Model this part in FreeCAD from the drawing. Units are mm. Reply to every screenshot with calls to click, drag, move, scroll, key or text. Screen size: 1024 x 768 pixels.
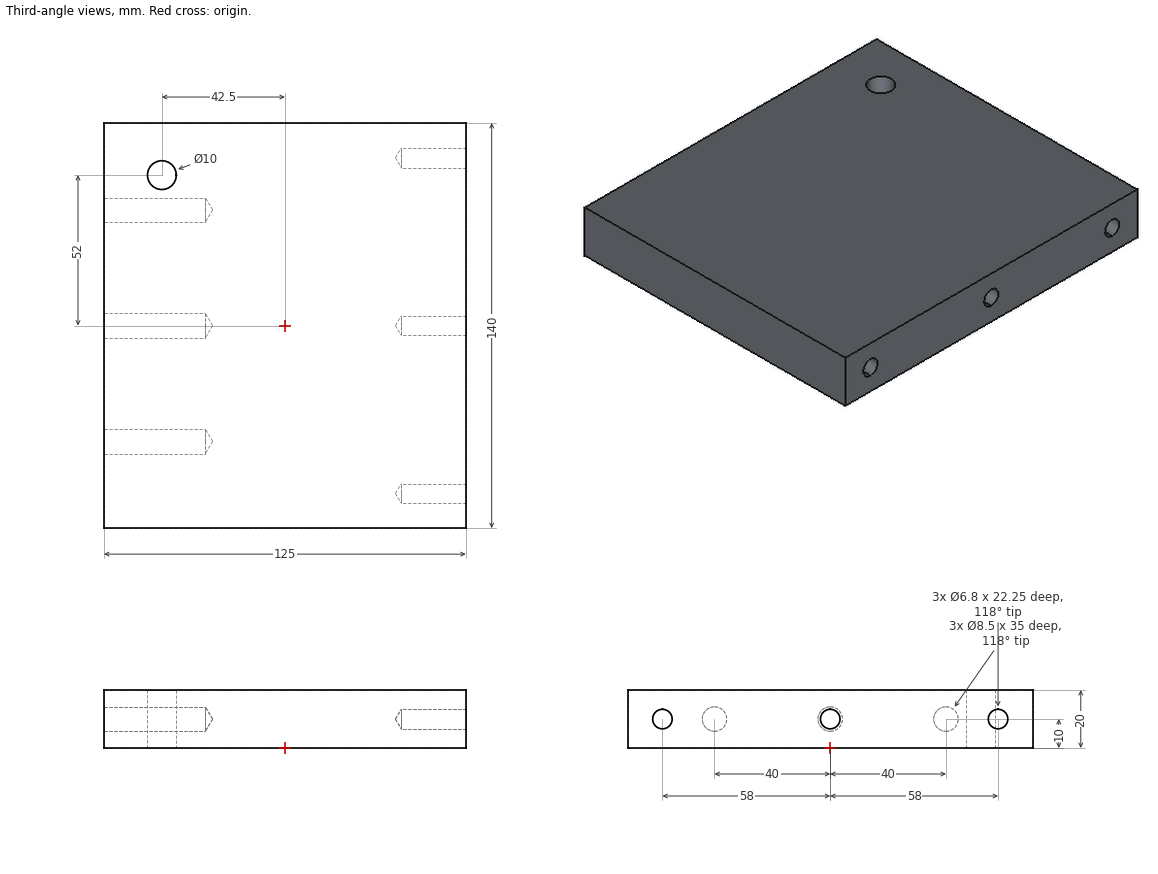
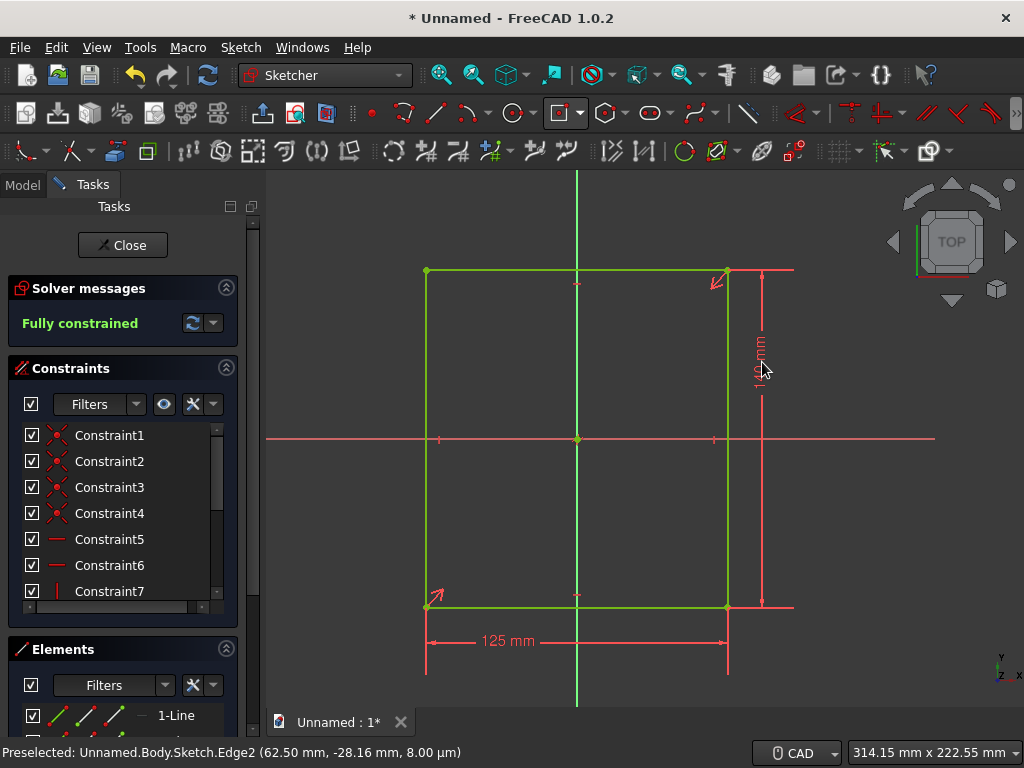
click(123, 245)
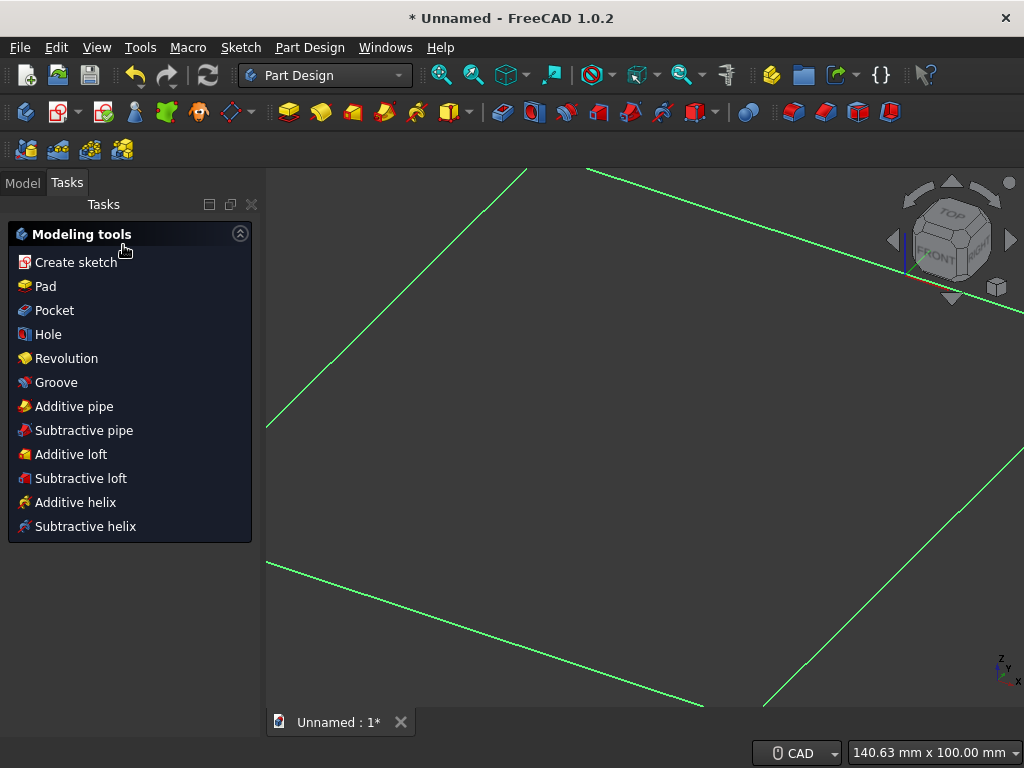
click(290, 112)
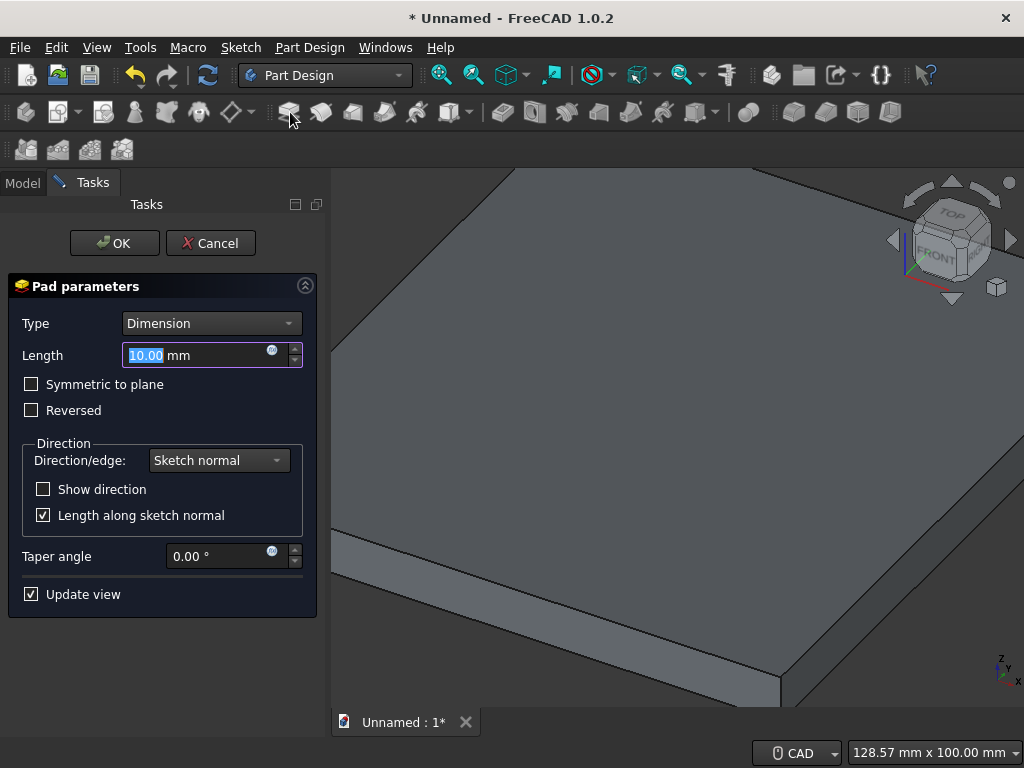
text(20)
key(Tab)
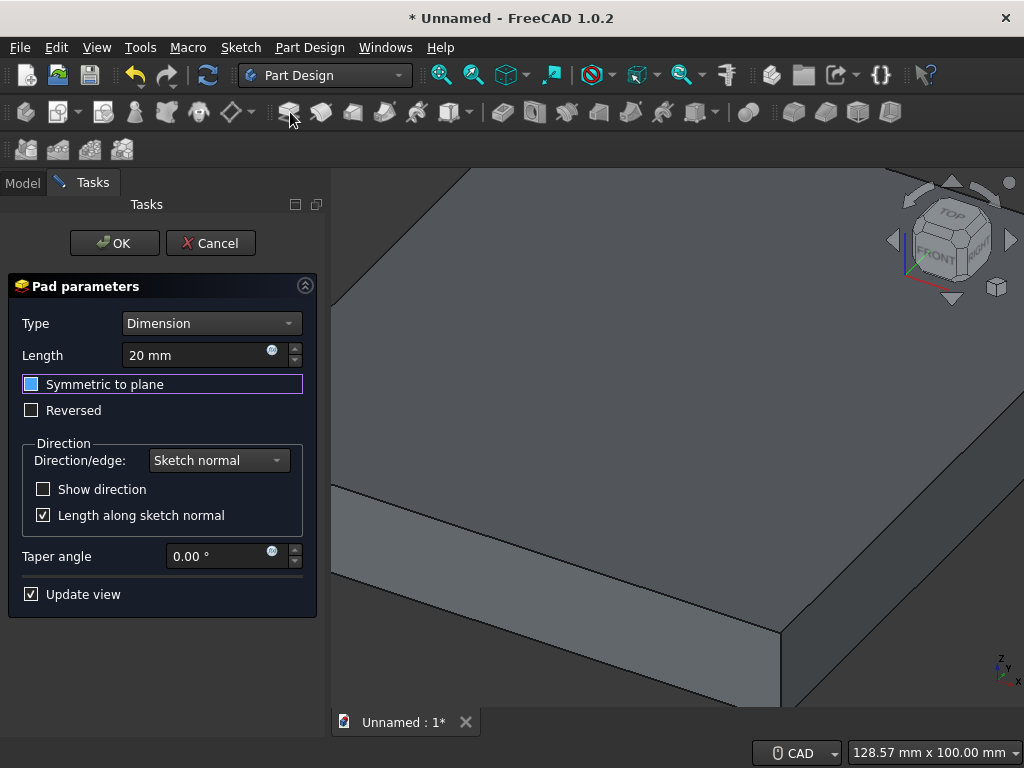
click(115, 243)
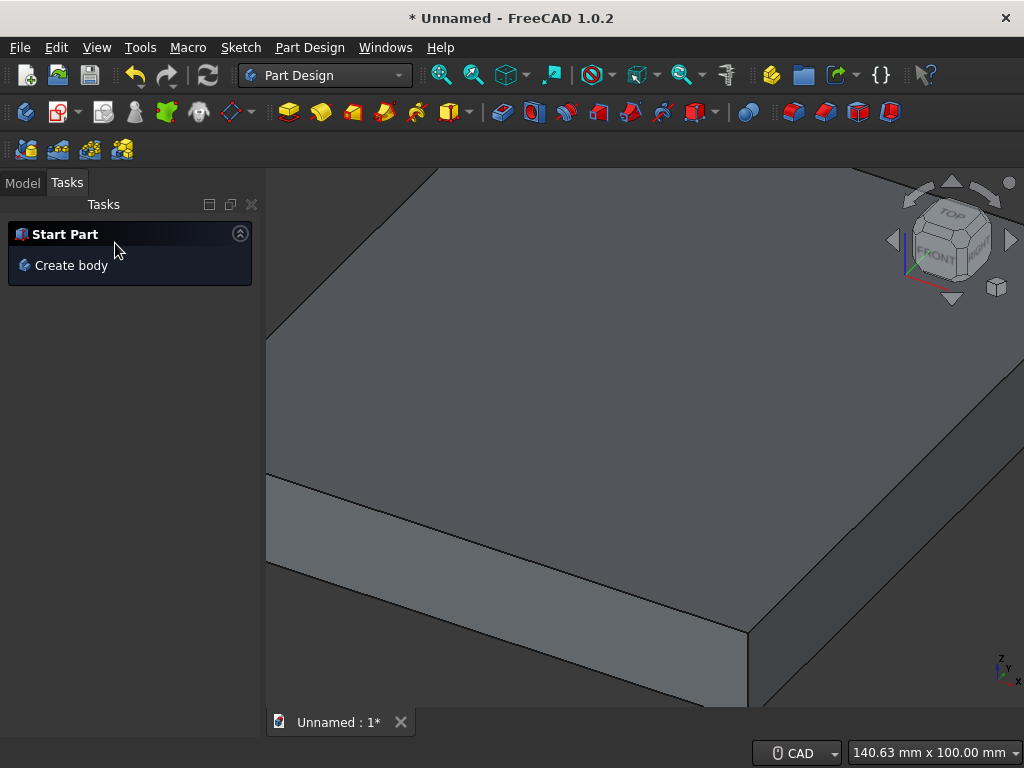
click(442, 76)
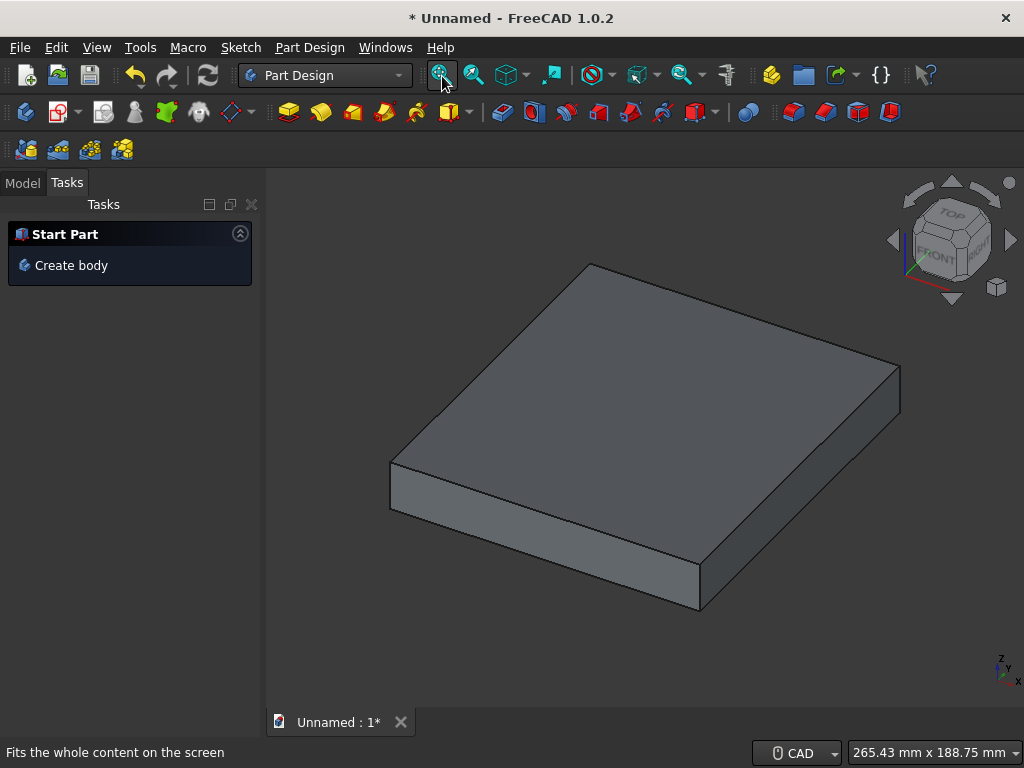
key(6)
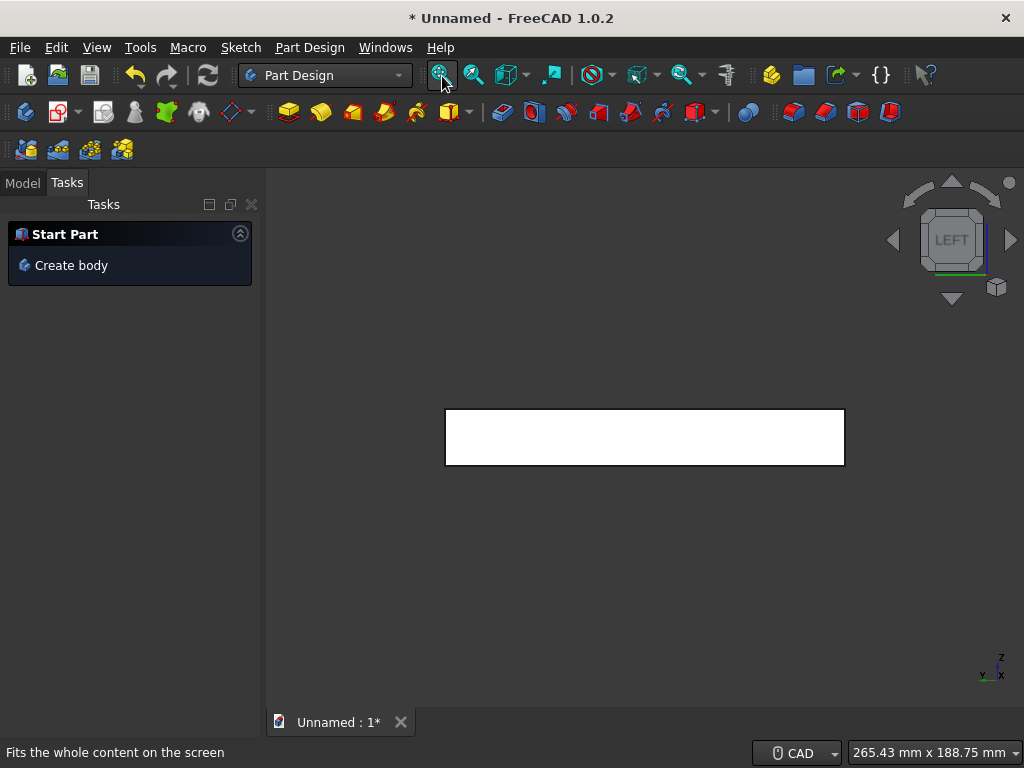
click(474, 436)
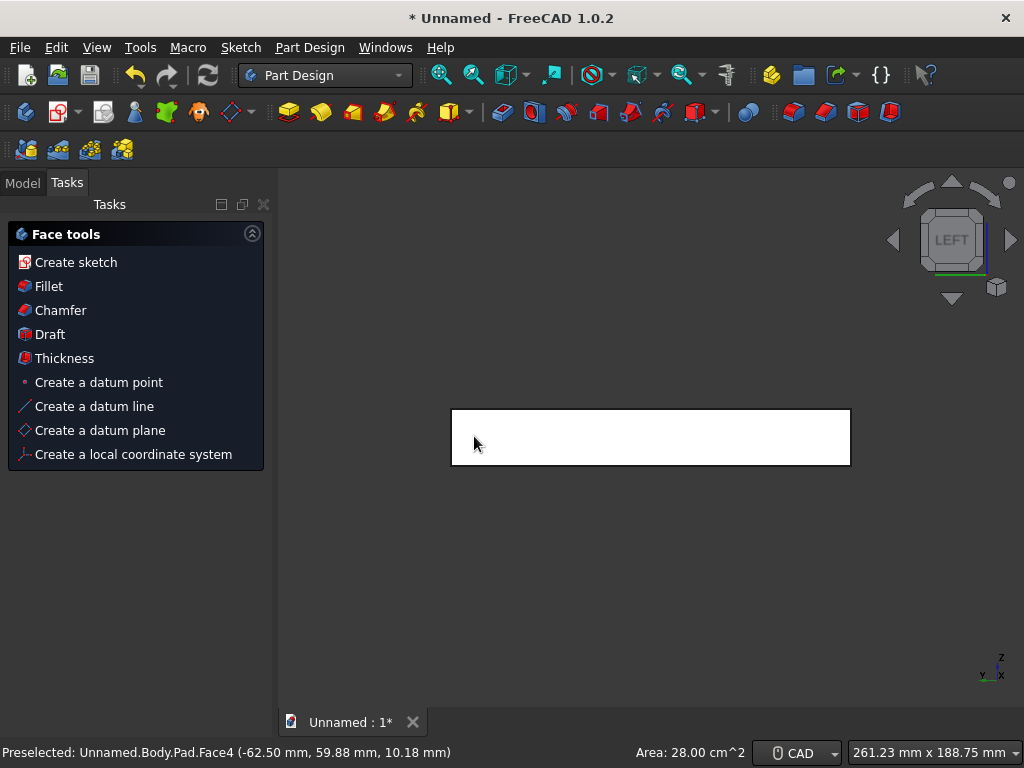
click(58, 112)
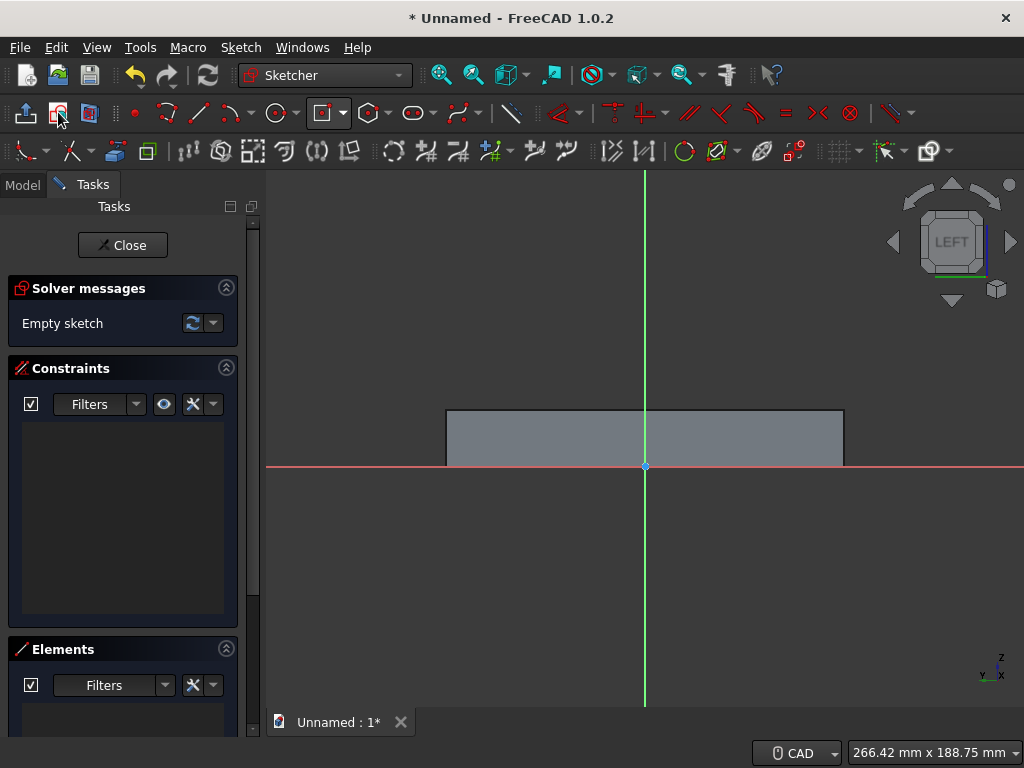
scroll(784, 463, up, 2)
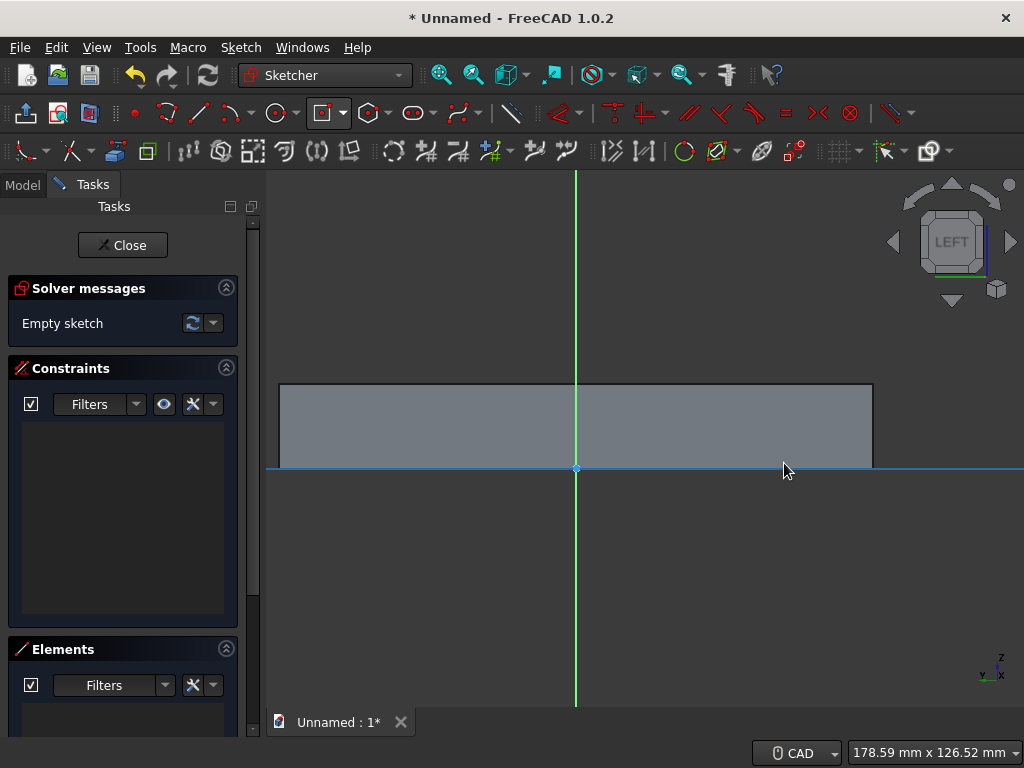
click(276, 114)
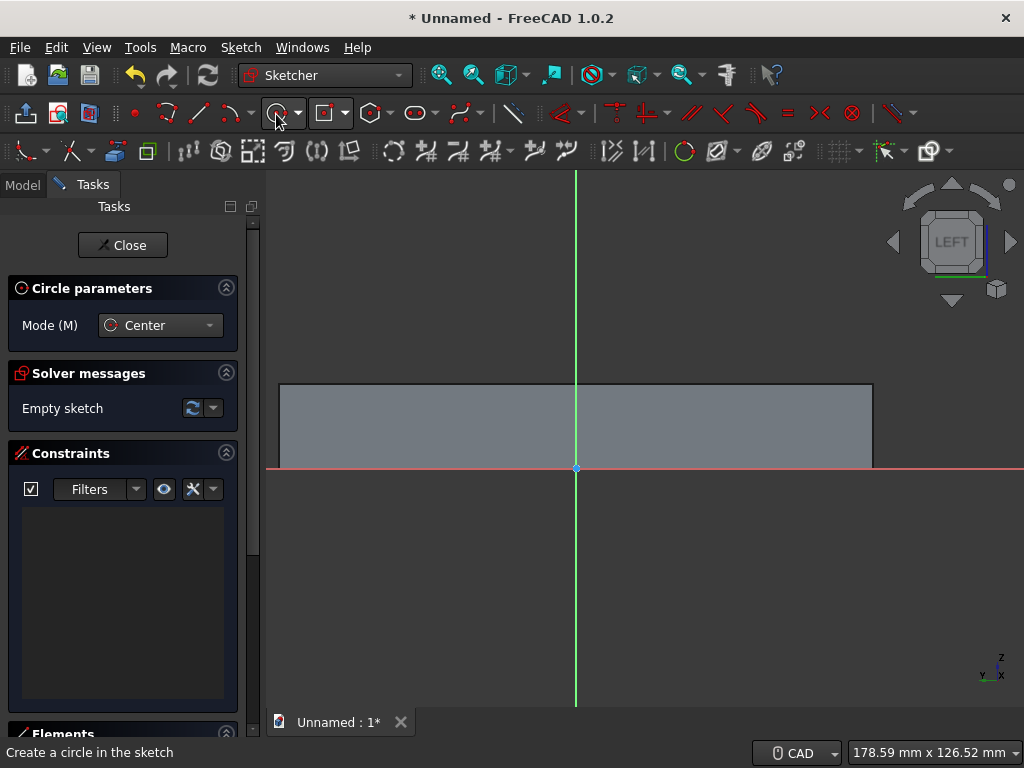
scroll(407, 426, up, 2)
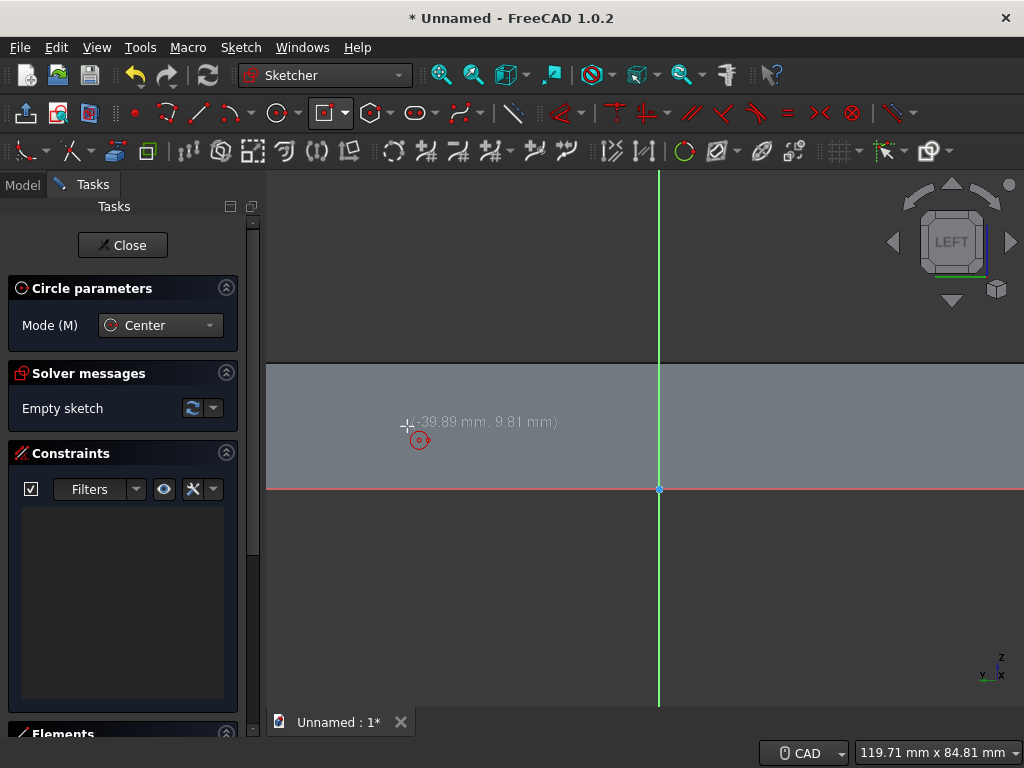
click(406, 426)
click(425, 407)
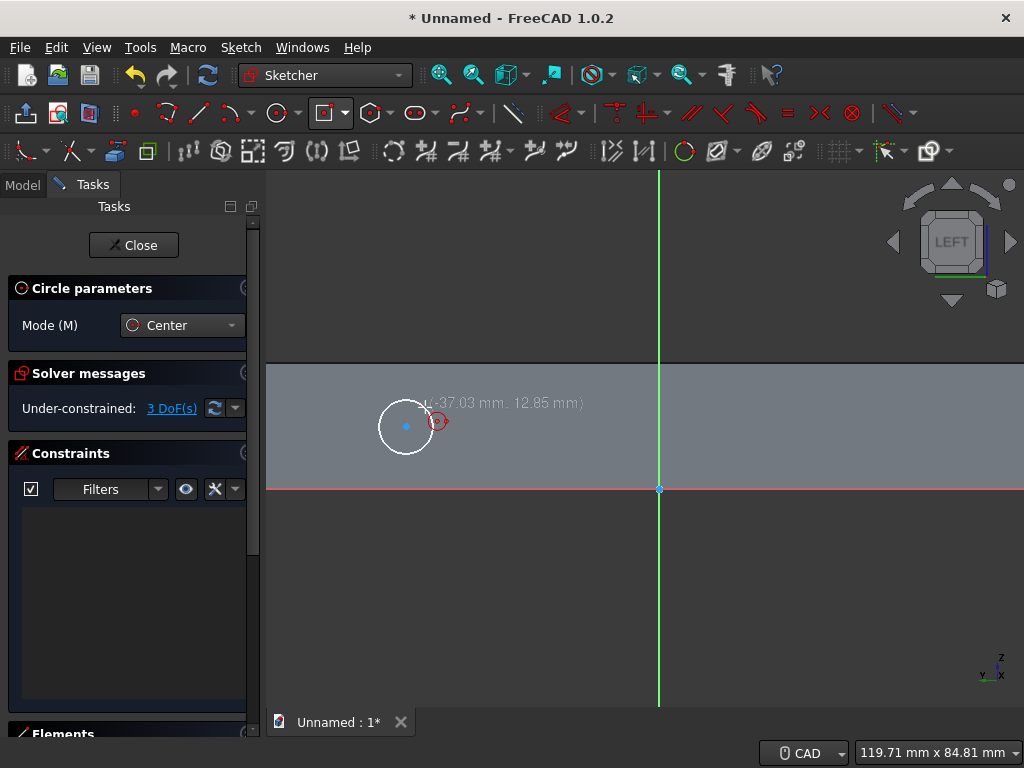
click(659, 426)
click(679, 407)